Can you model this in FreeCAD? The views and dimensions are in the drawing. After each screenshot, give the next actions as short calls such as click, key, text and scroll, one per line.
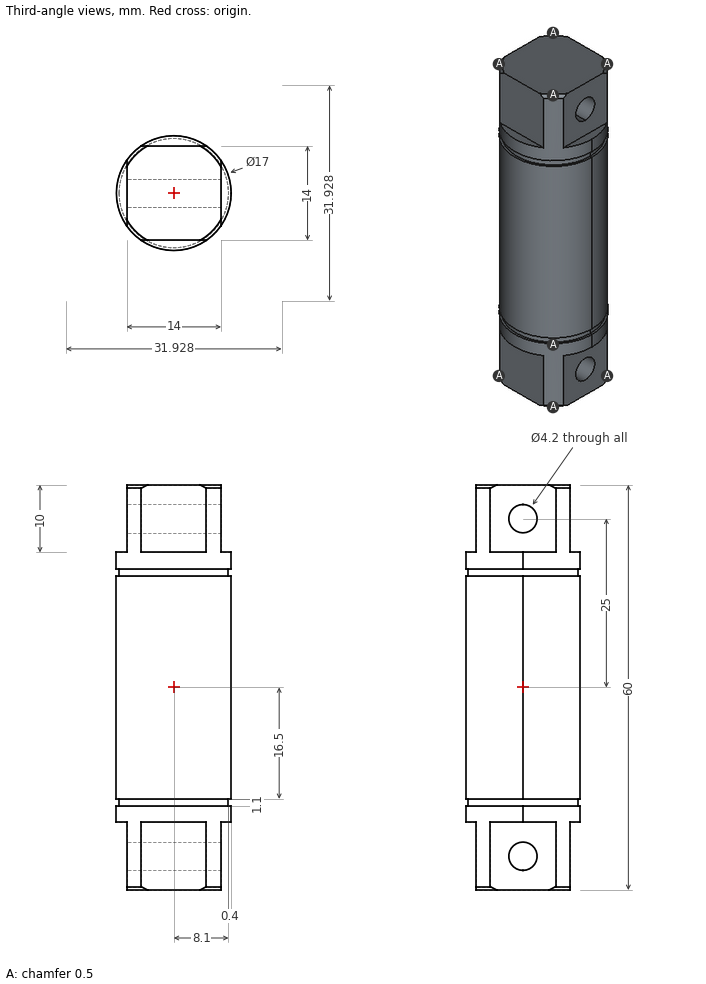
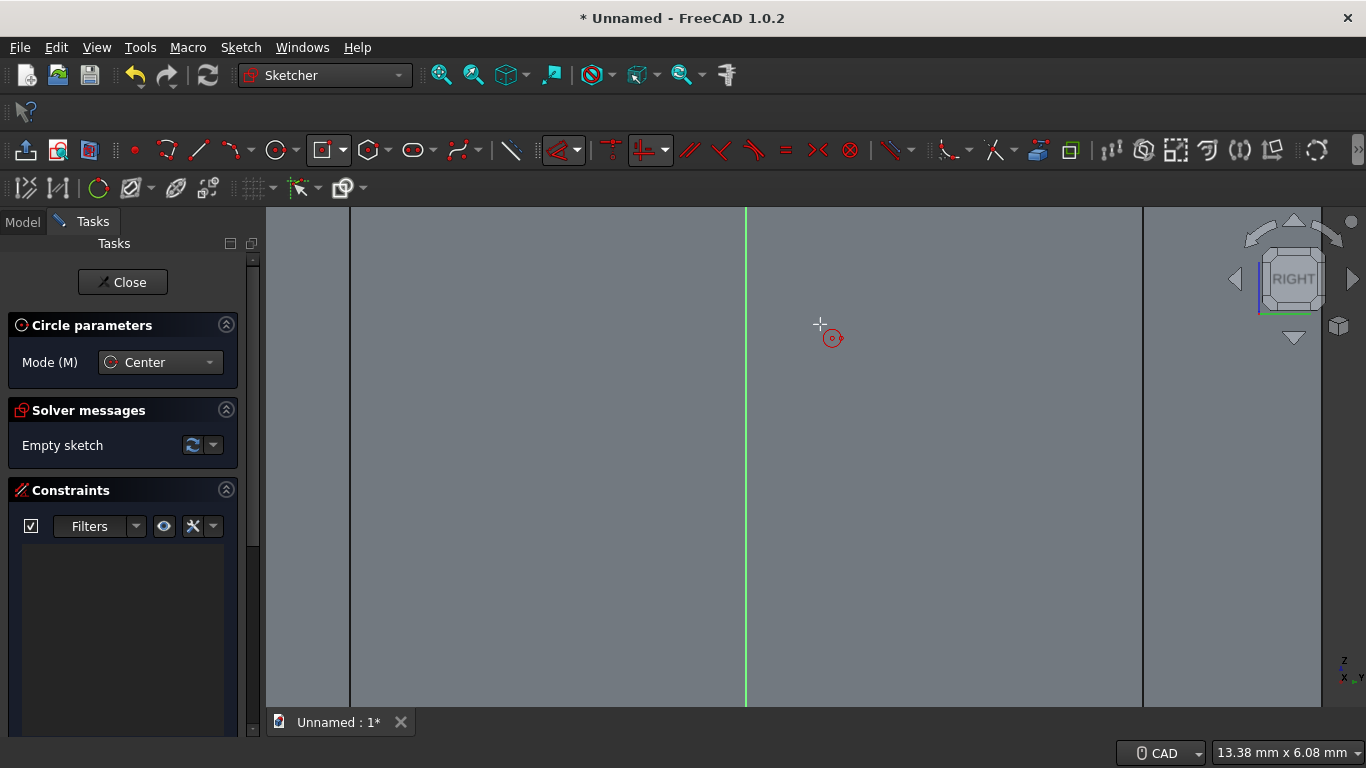
click(746, 452)
move(869, 330)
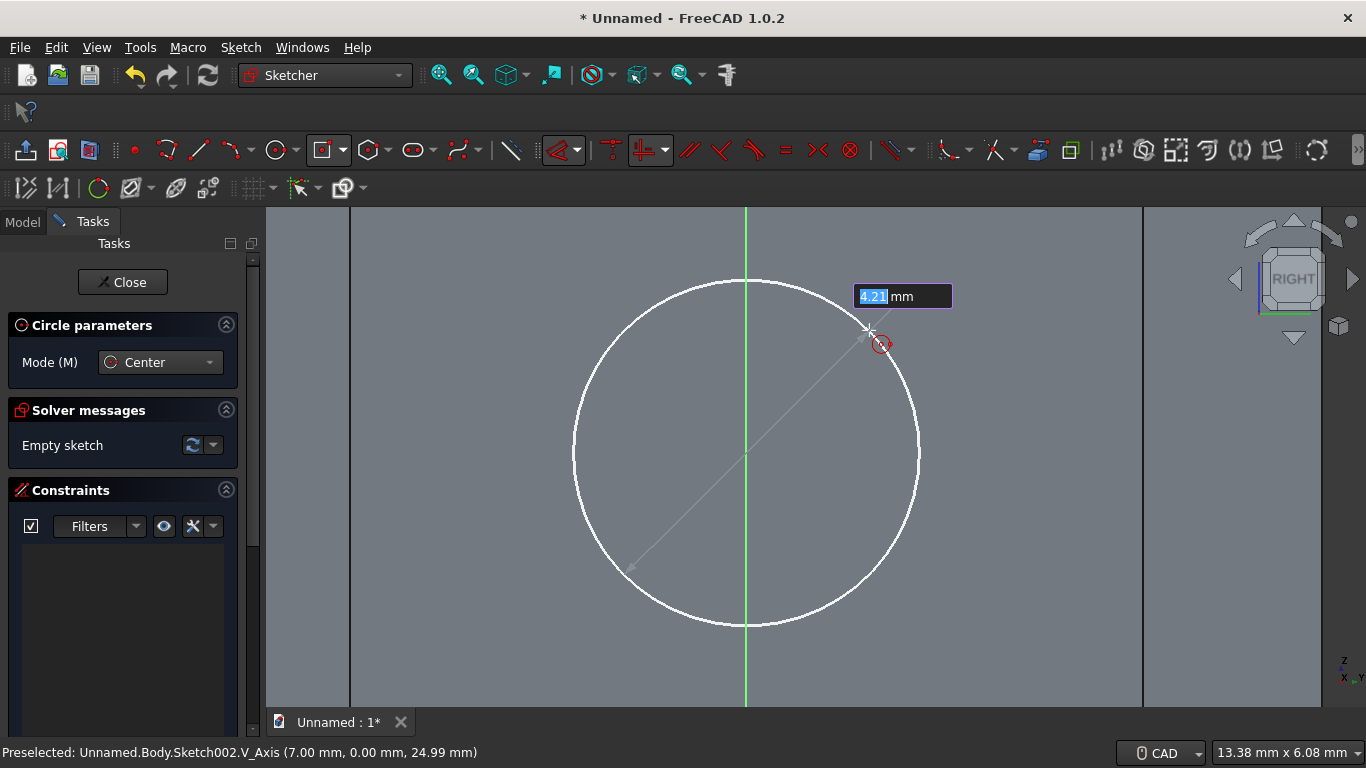
text(4.2)
key(Return)
key(Escape)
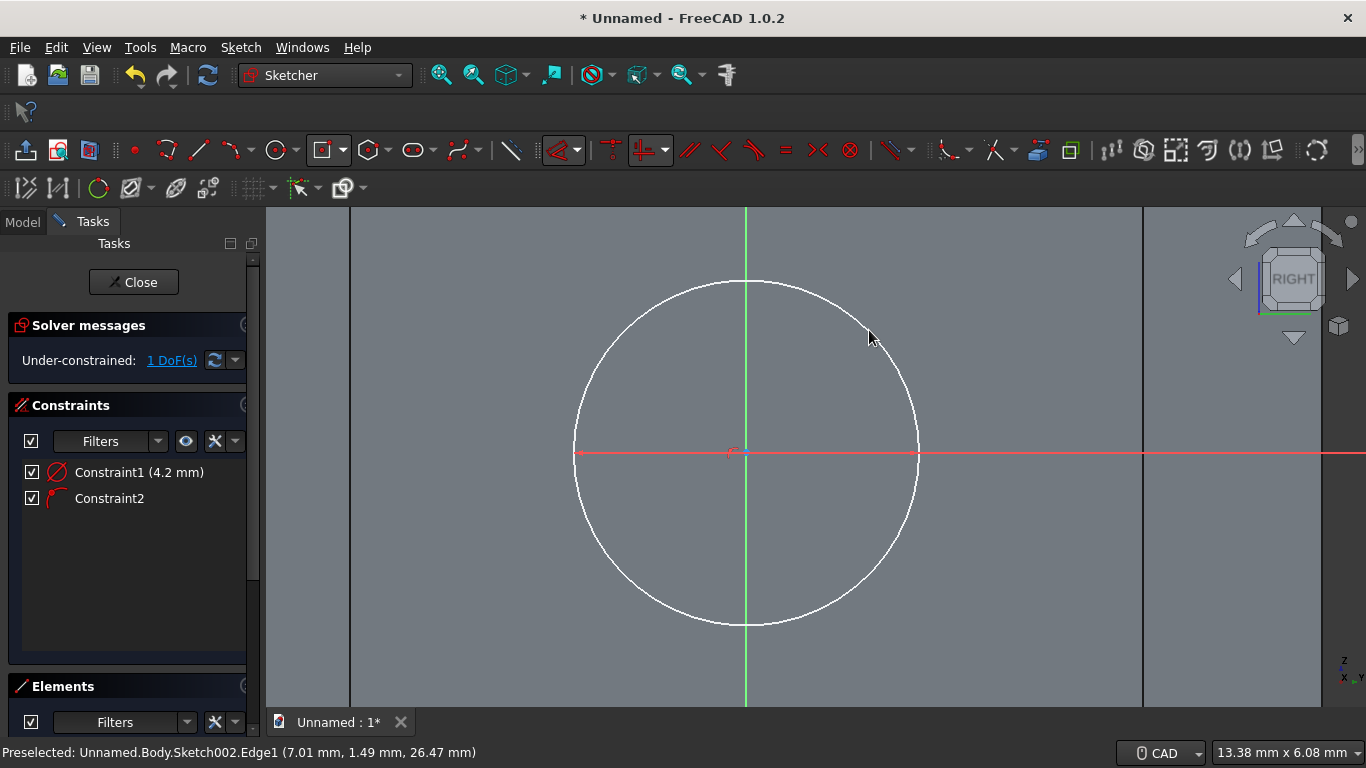
click(746, 453)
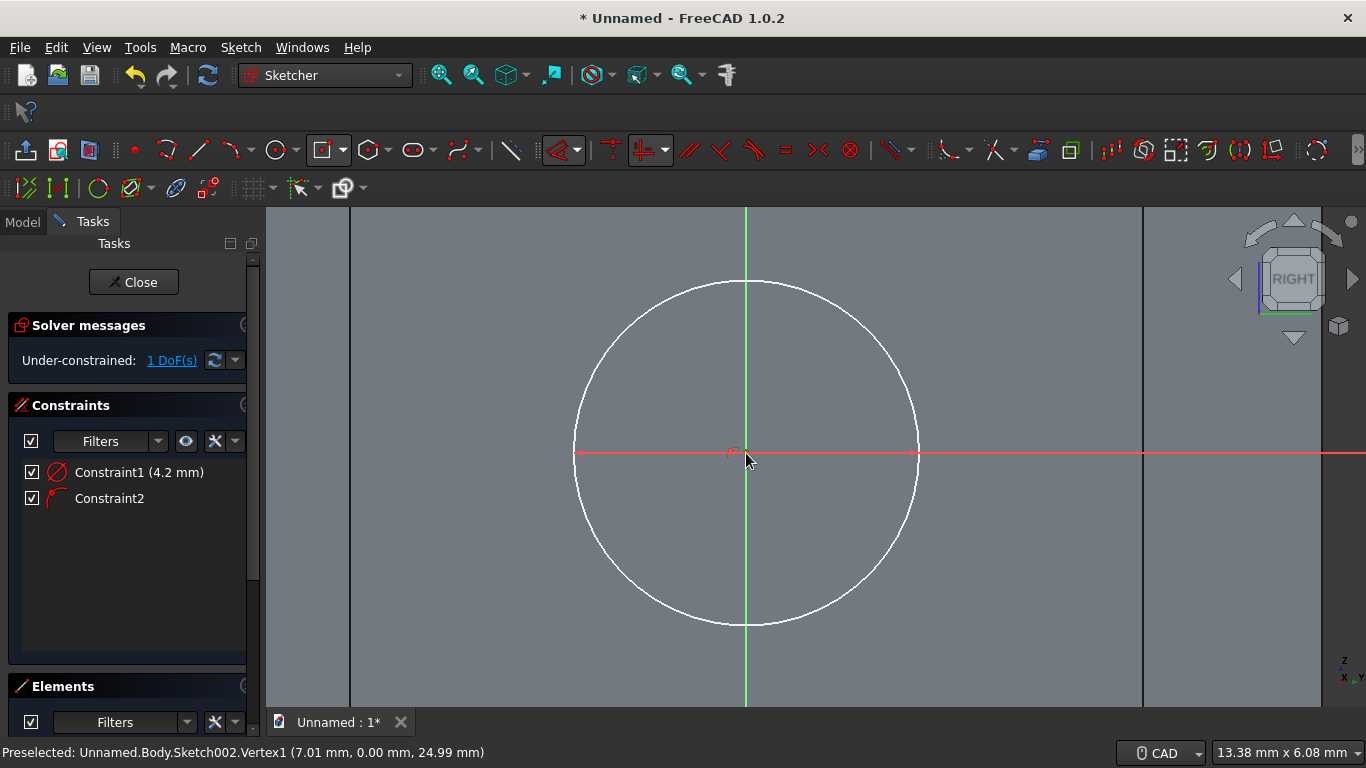
key(i)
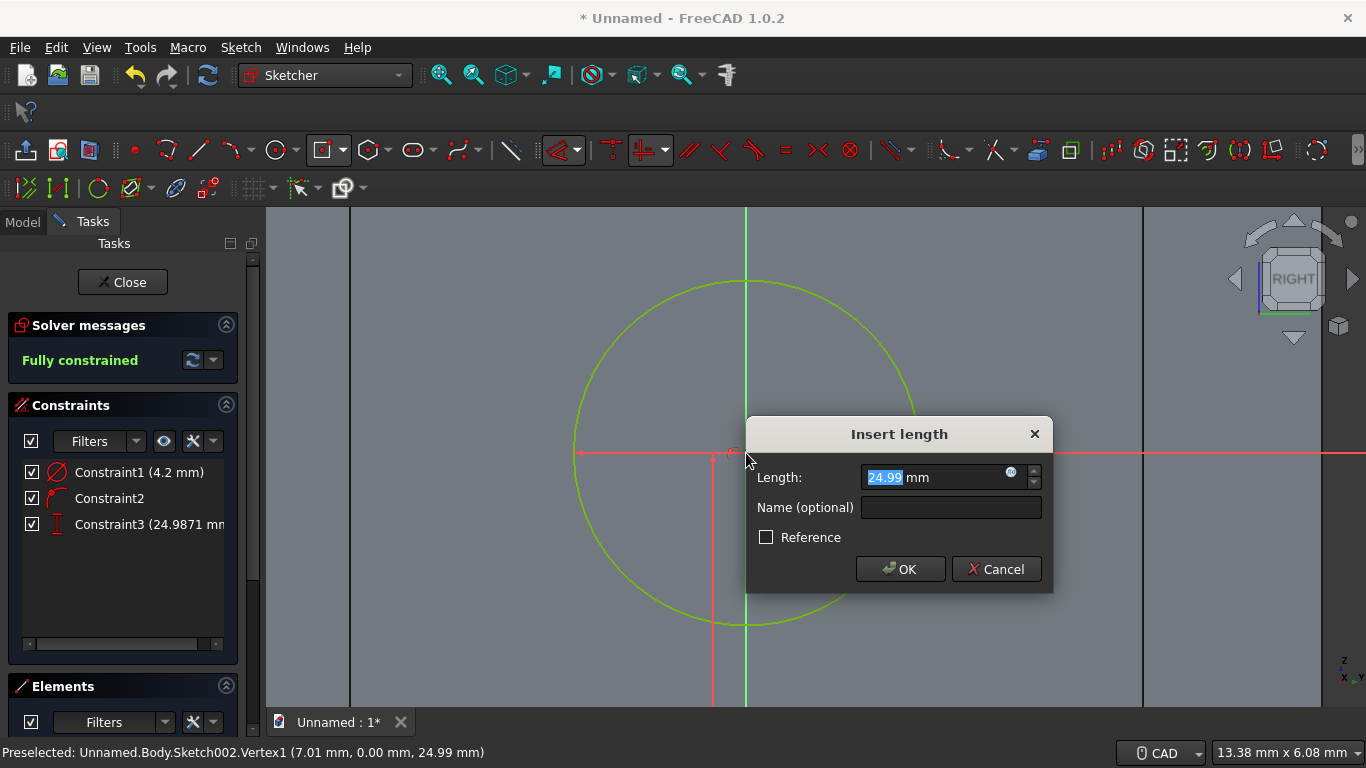
text(25)
key(Return)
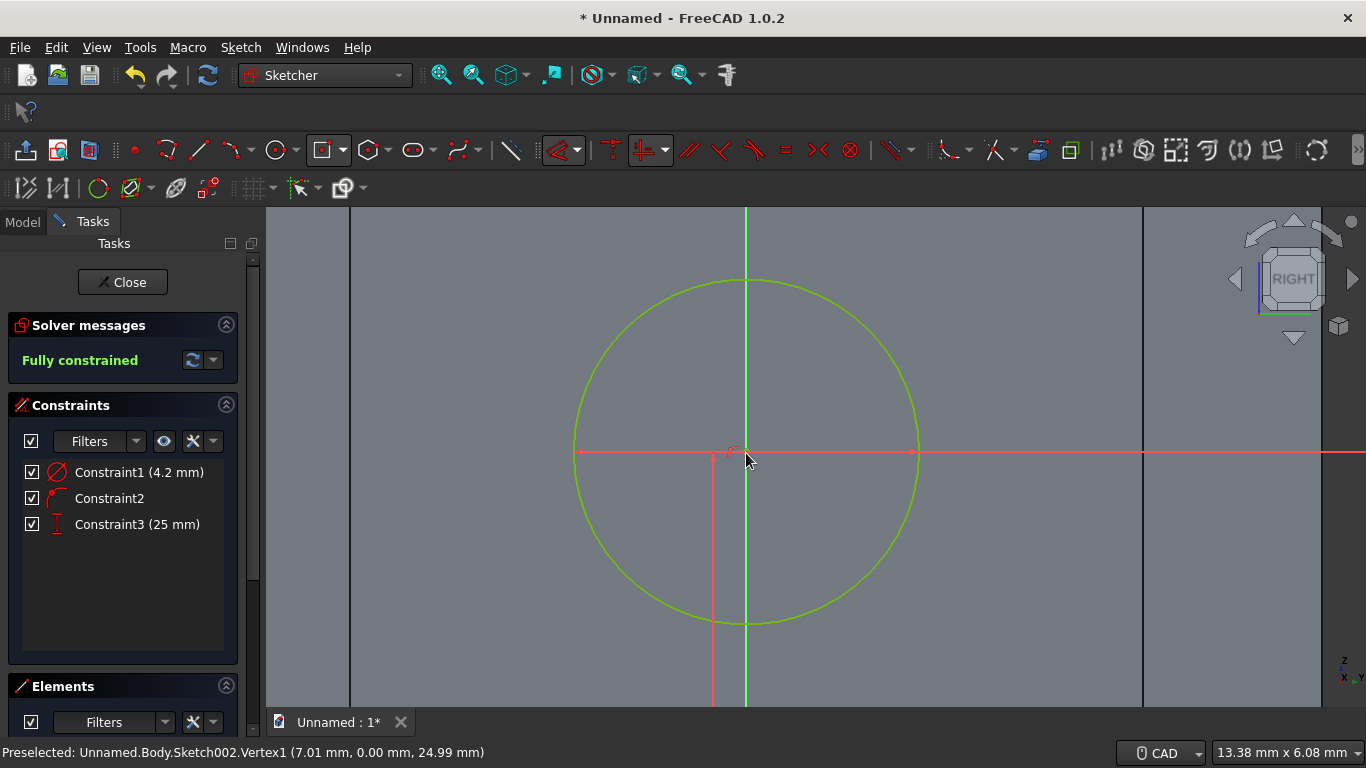
click(123, 282)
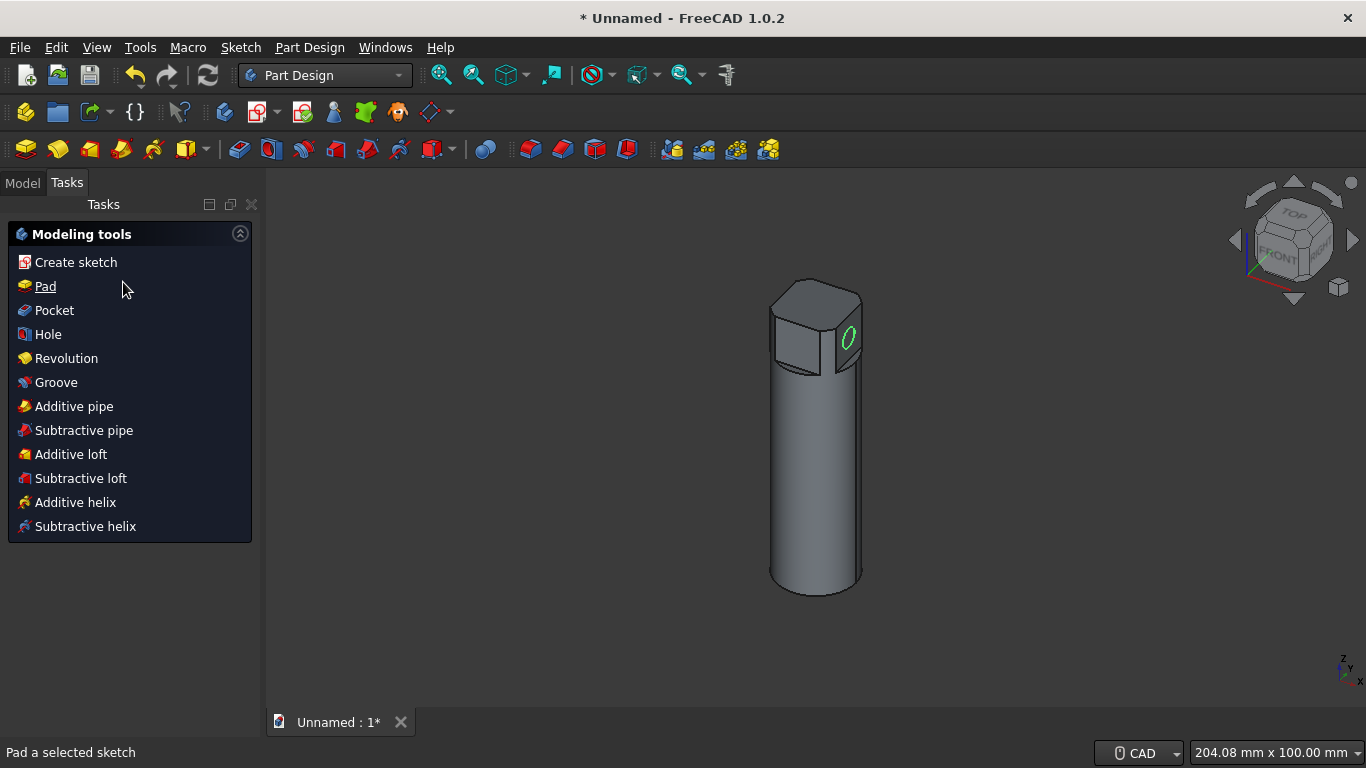
click(272, 150)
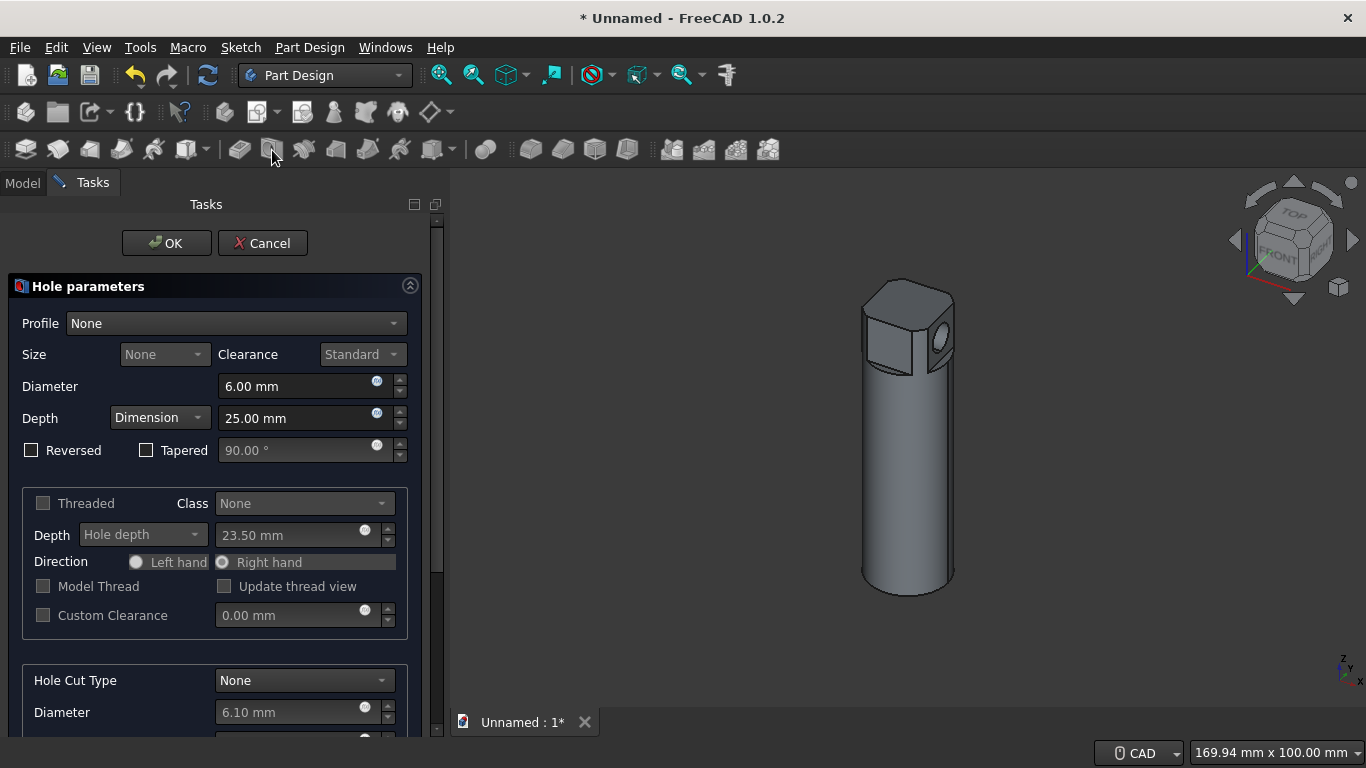
triple_click(305, 386)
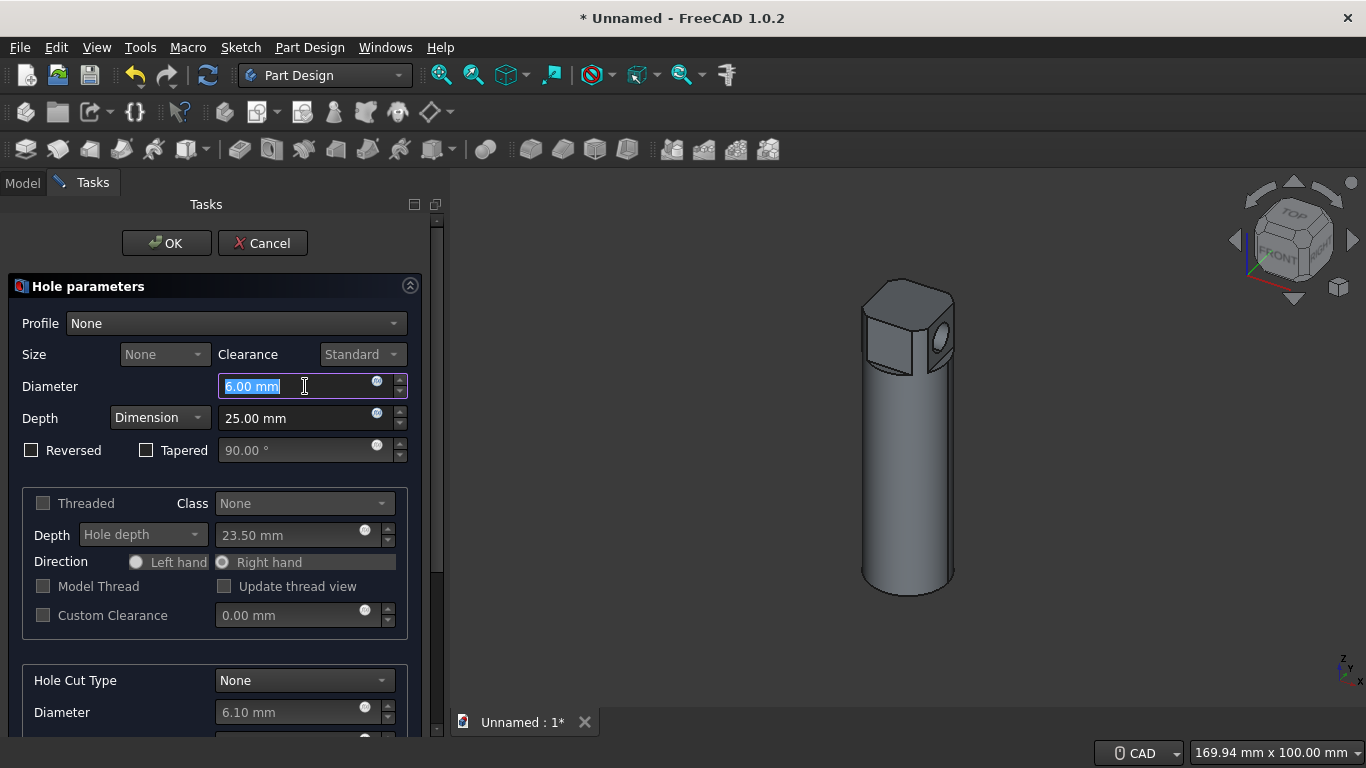
text(4.2)
key(Tab)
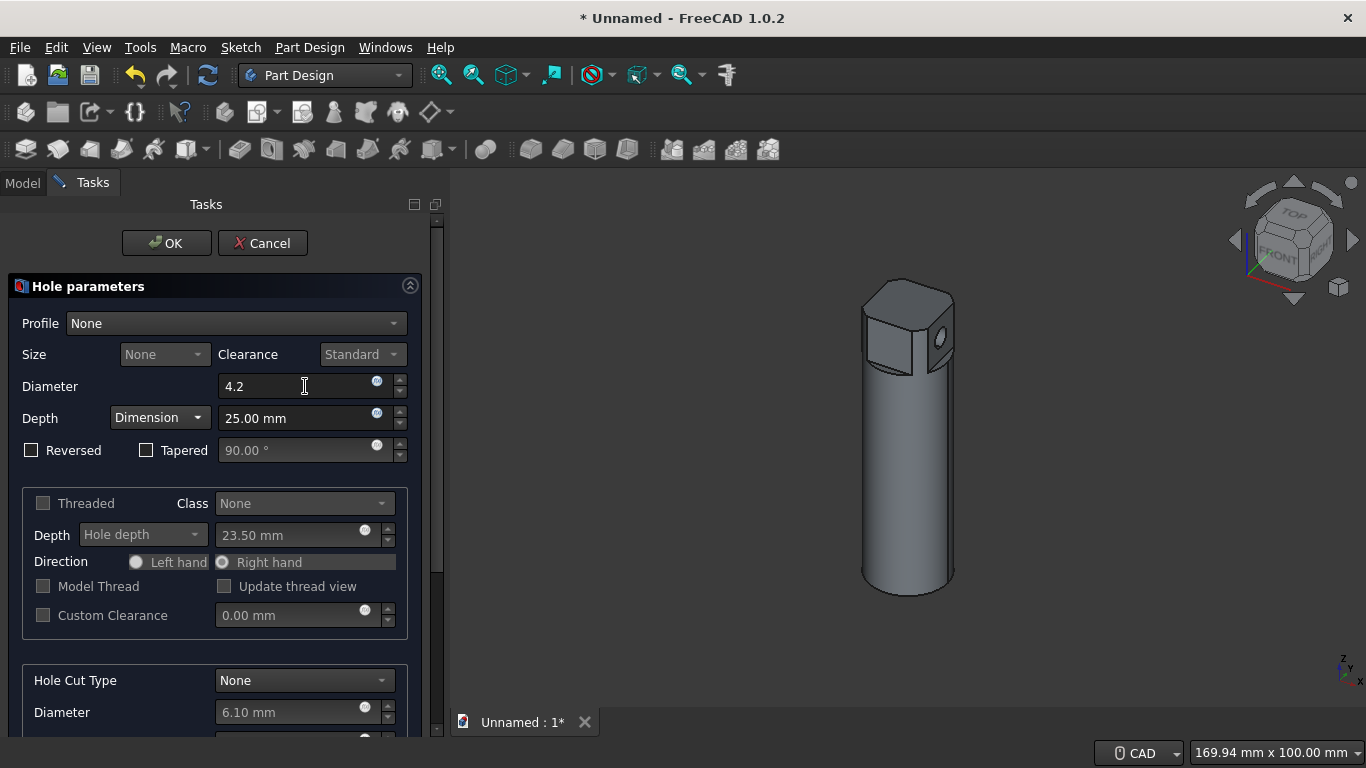
click(161, 418)